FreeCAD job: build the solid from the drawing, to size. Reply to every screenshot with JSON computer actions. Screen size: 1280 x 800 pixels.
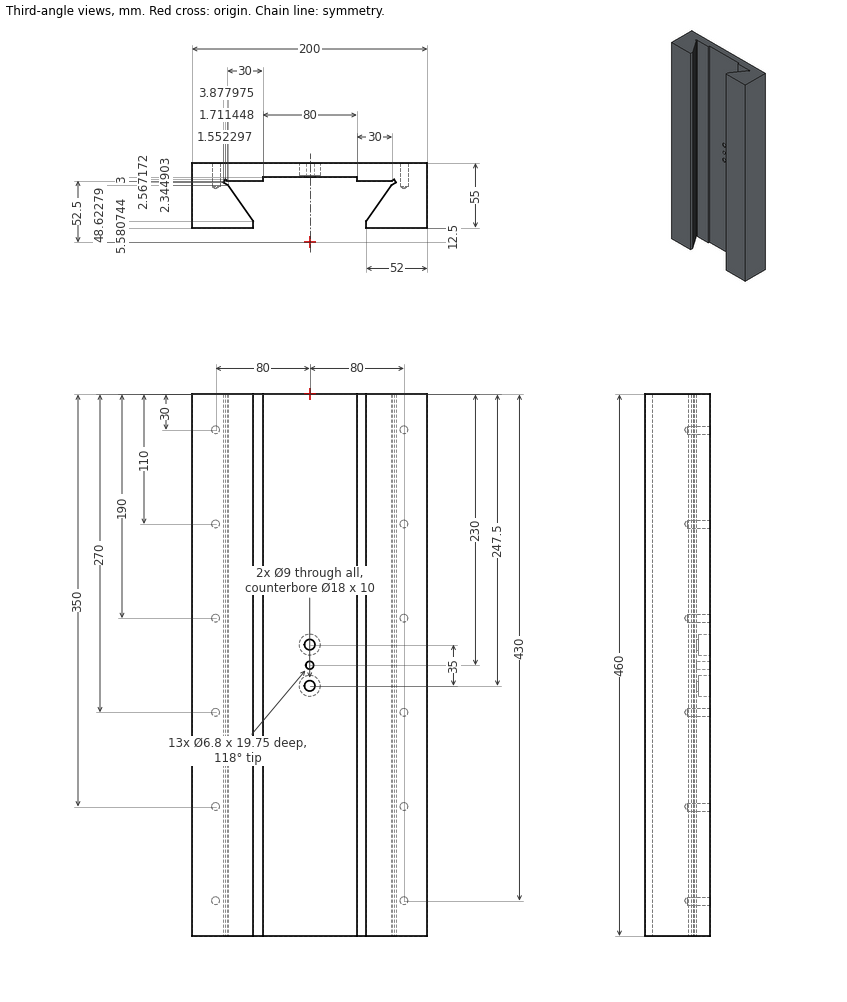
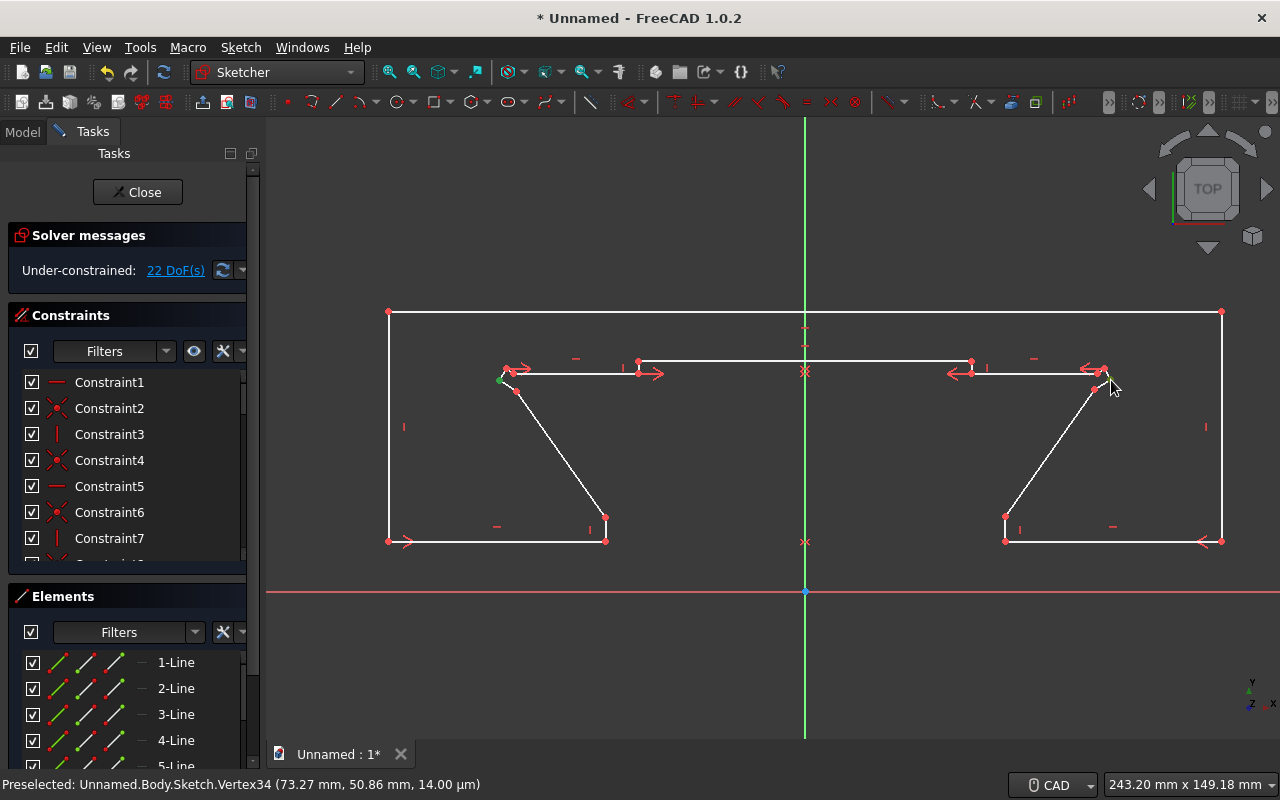
{"action": "left_click", "coordinate": [805, 671]}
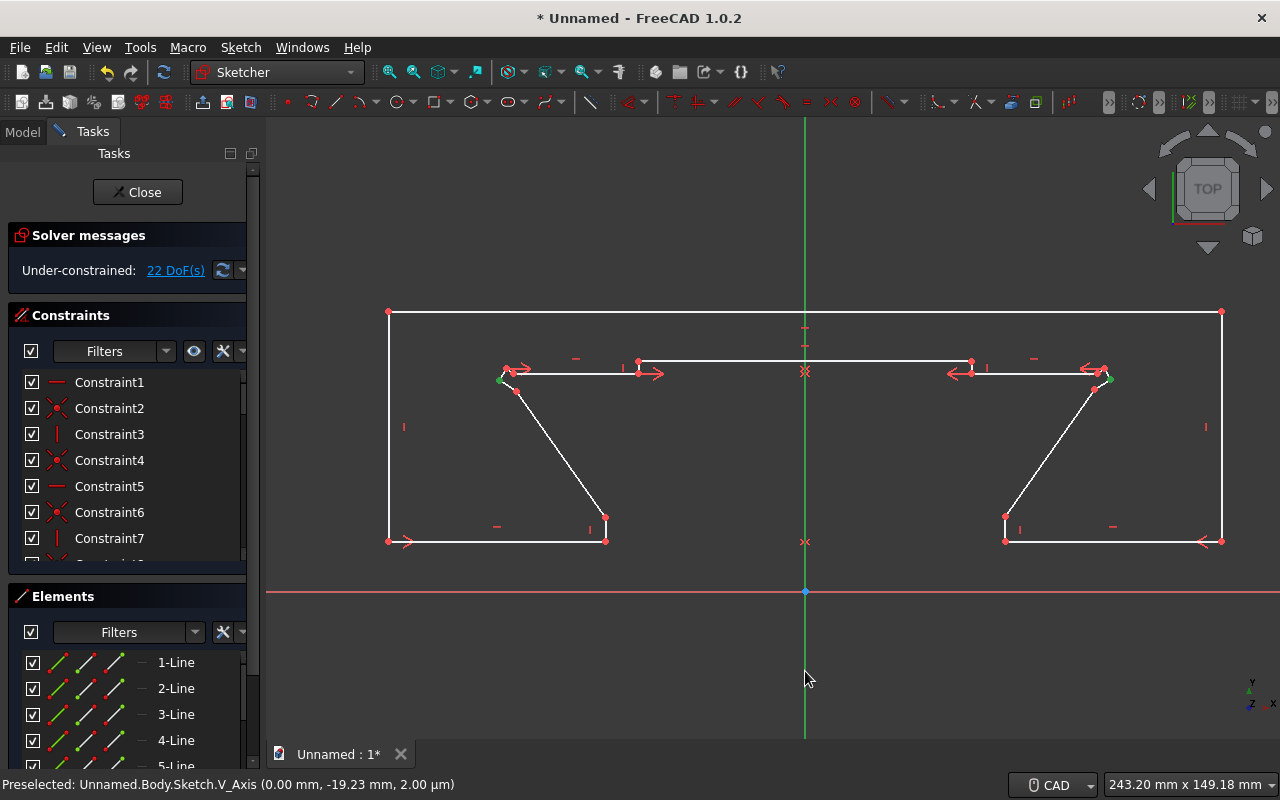
{"action": "left_click", "coordinate": [832, 102]}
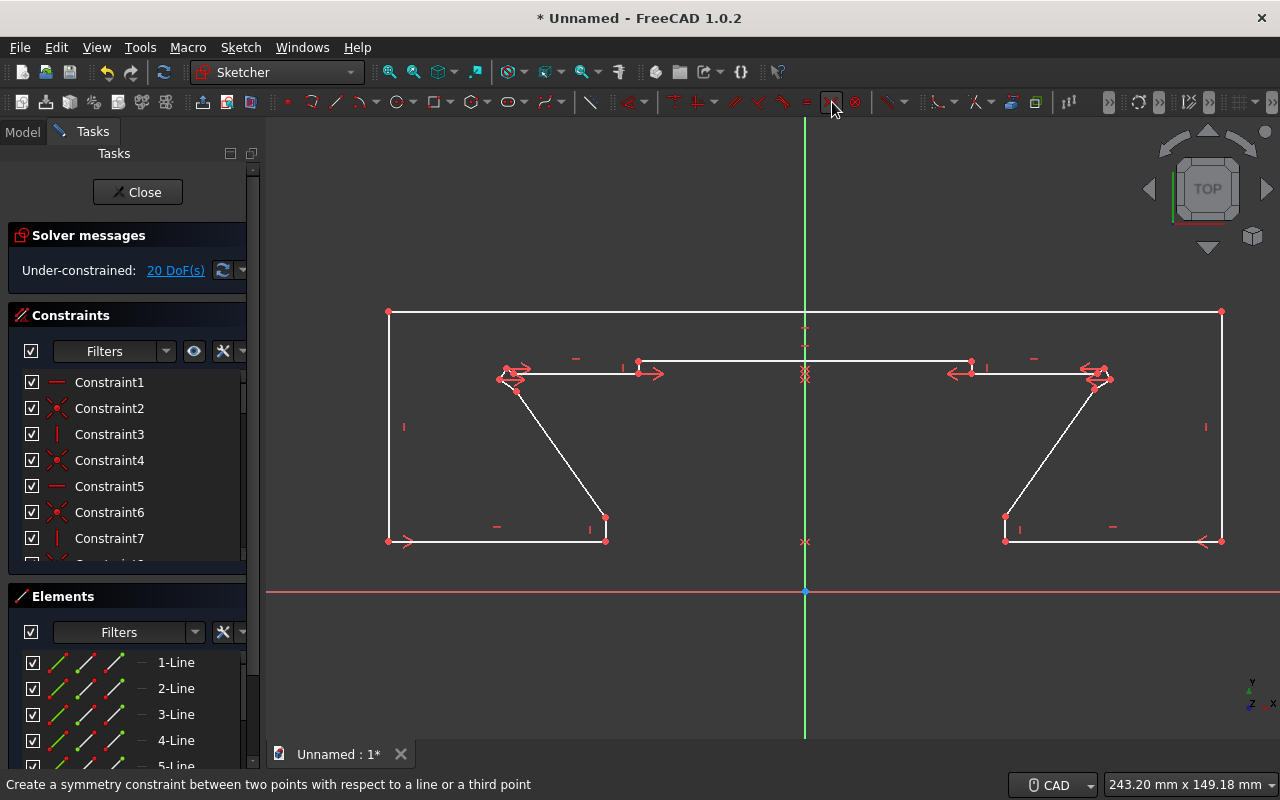
{"action": "left_click", "coordinate": [516, 391]}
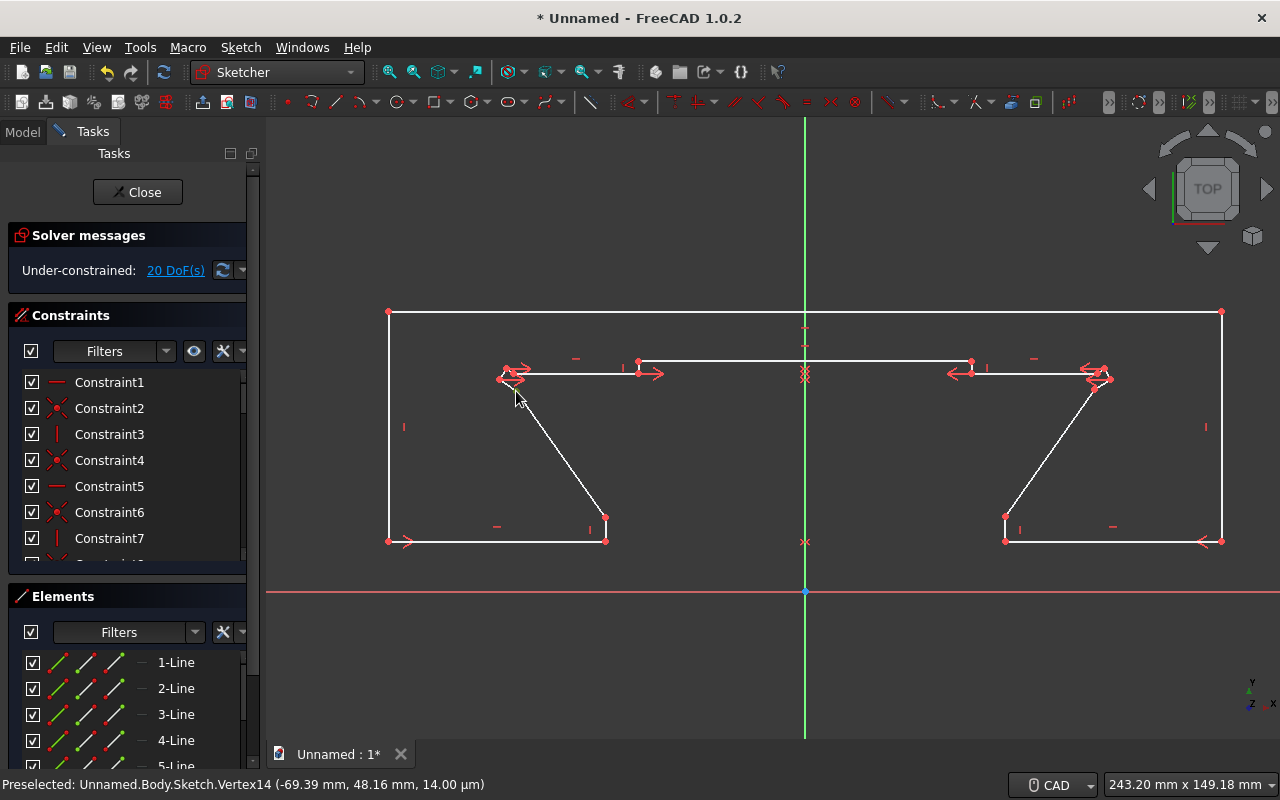
{"action": "left_click", "coordinate": [1095, 390]}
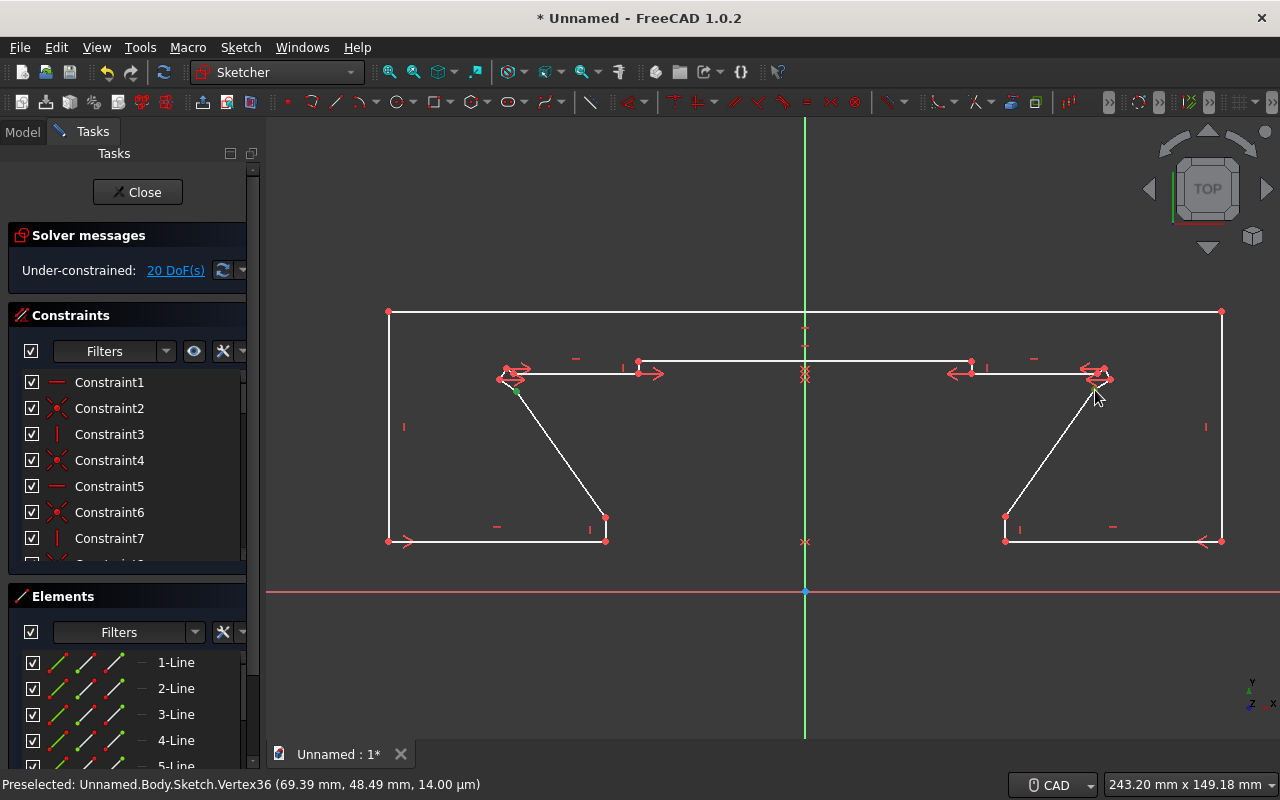
{"action": "left_click", "coordinate": [805, 671]}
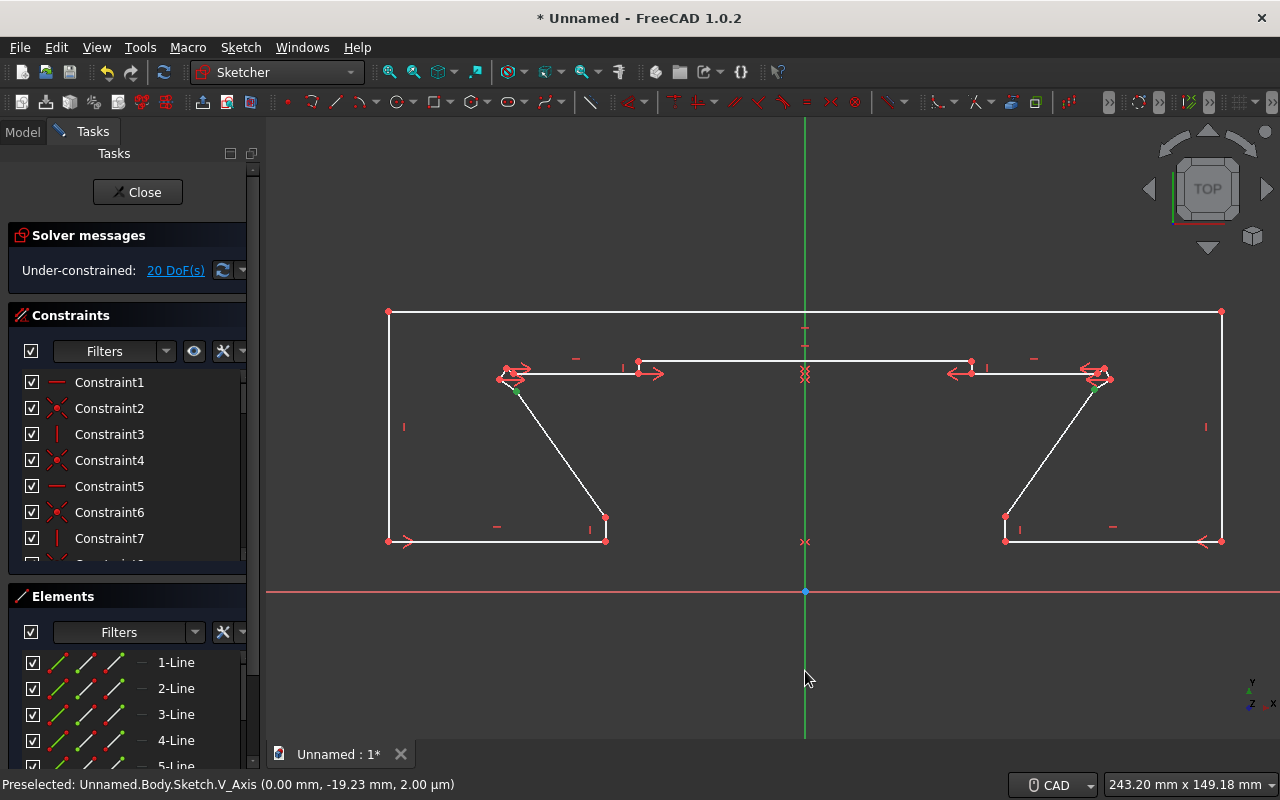
{"action": "left_click", "coordinate": [832, 102]}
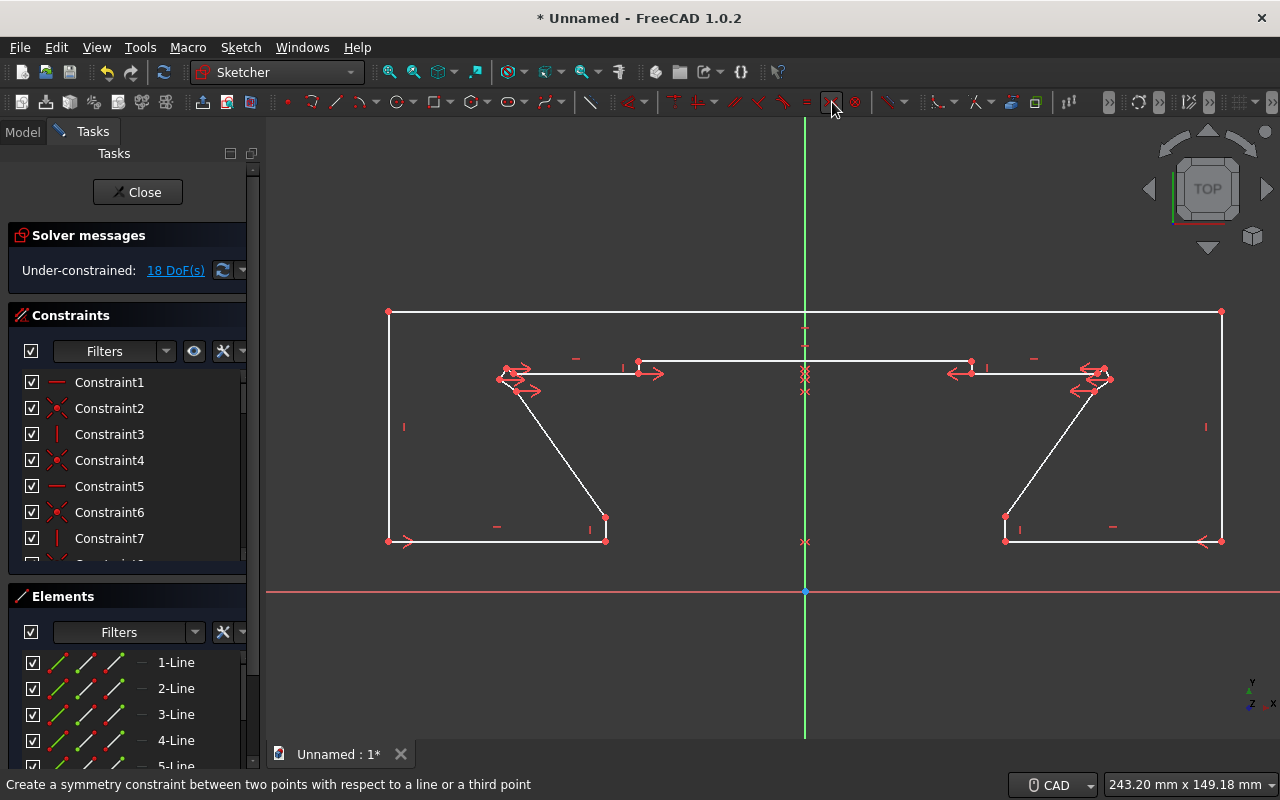
{"action": "left_click", "coordinate": [606, 518]}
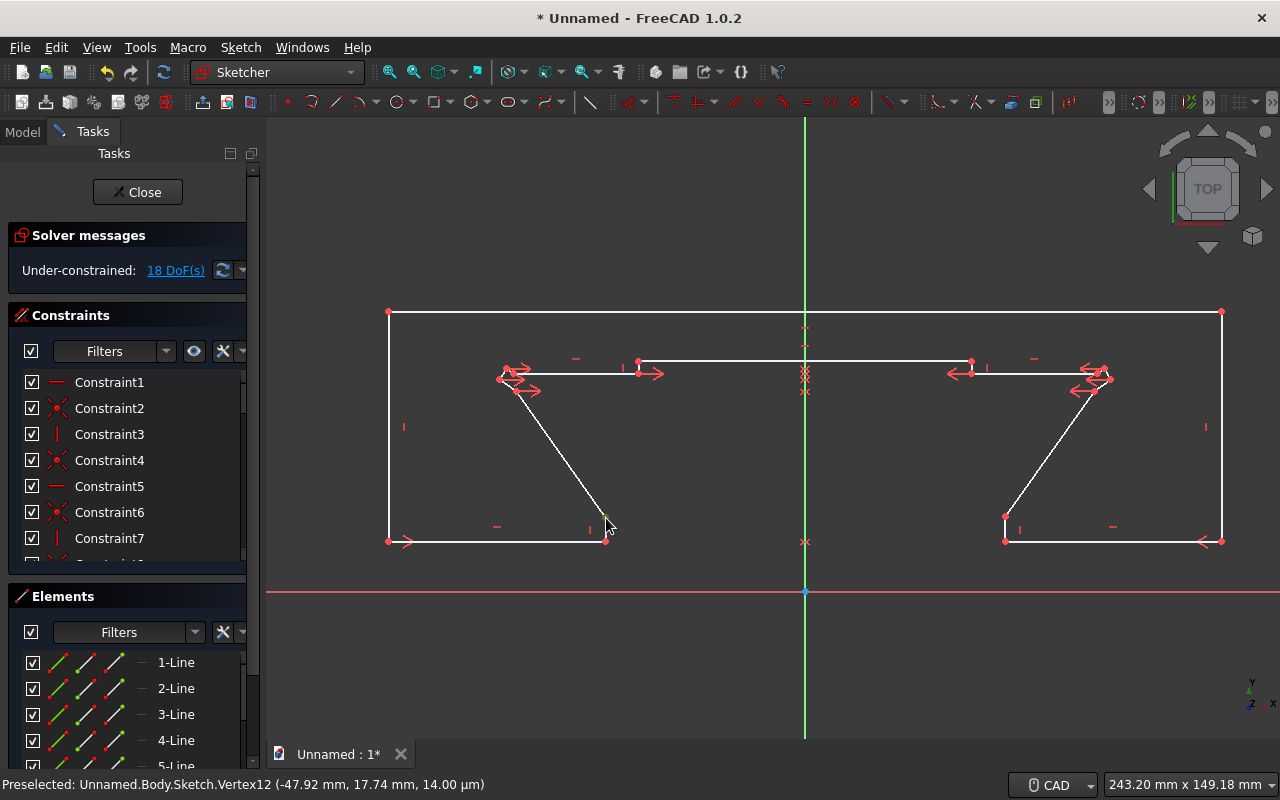
{"action": "left_click", "coordinate": [1005, 517]}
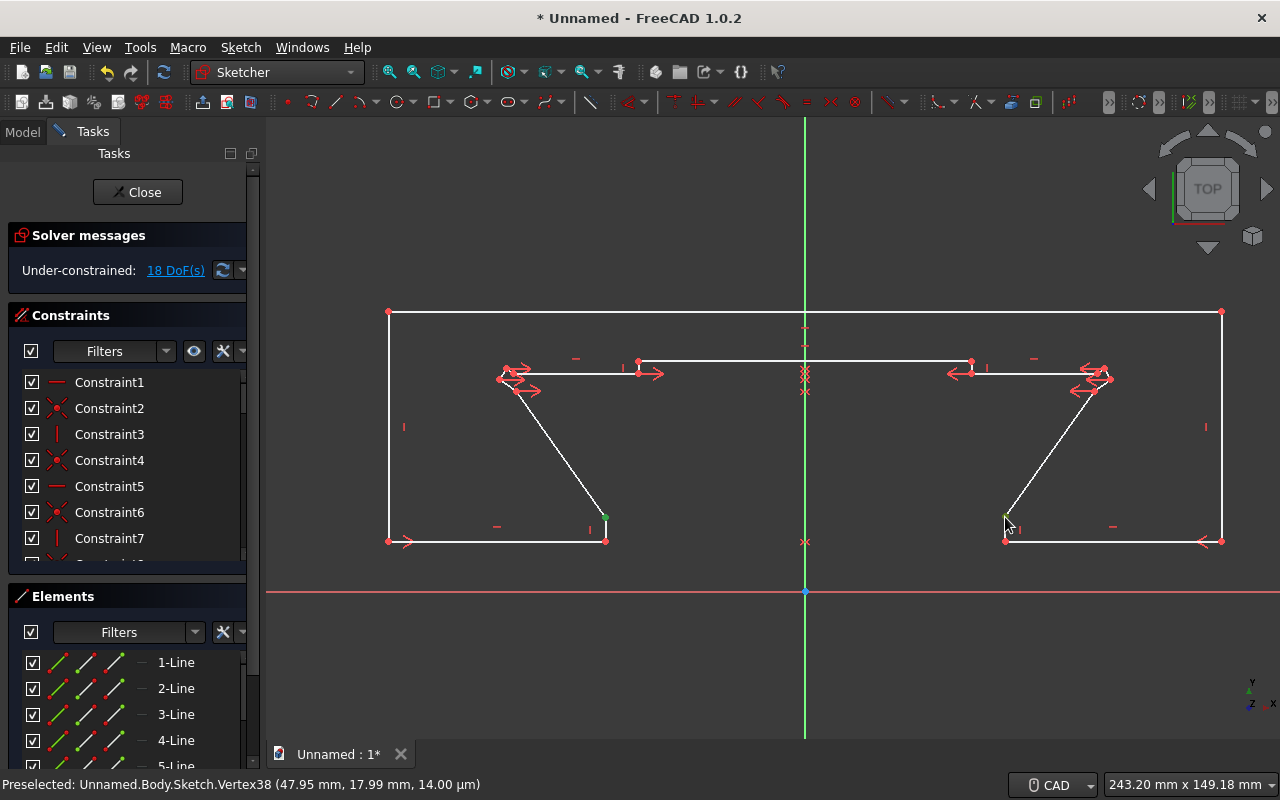
{"action": "left_click", "coordinate": [805, 671]}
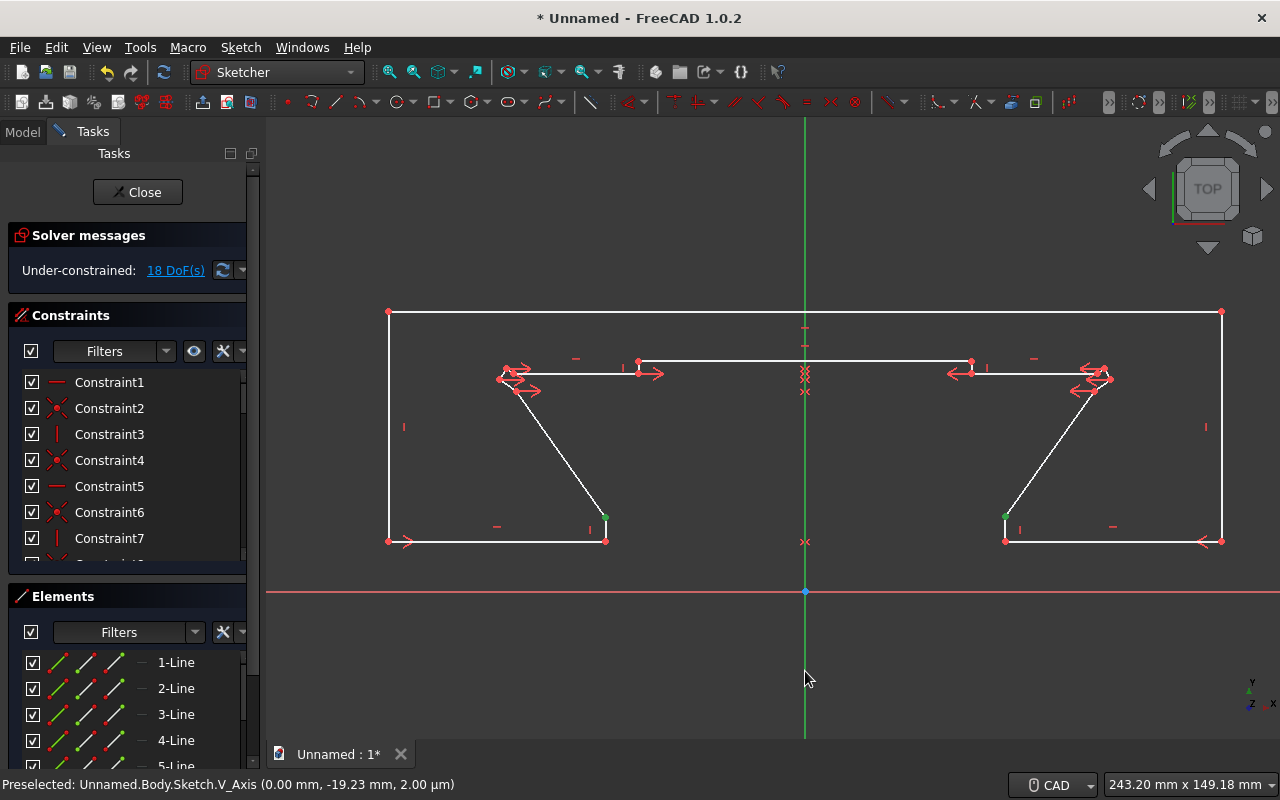
{"action": "left_click", "coordinate": [832, 102]}